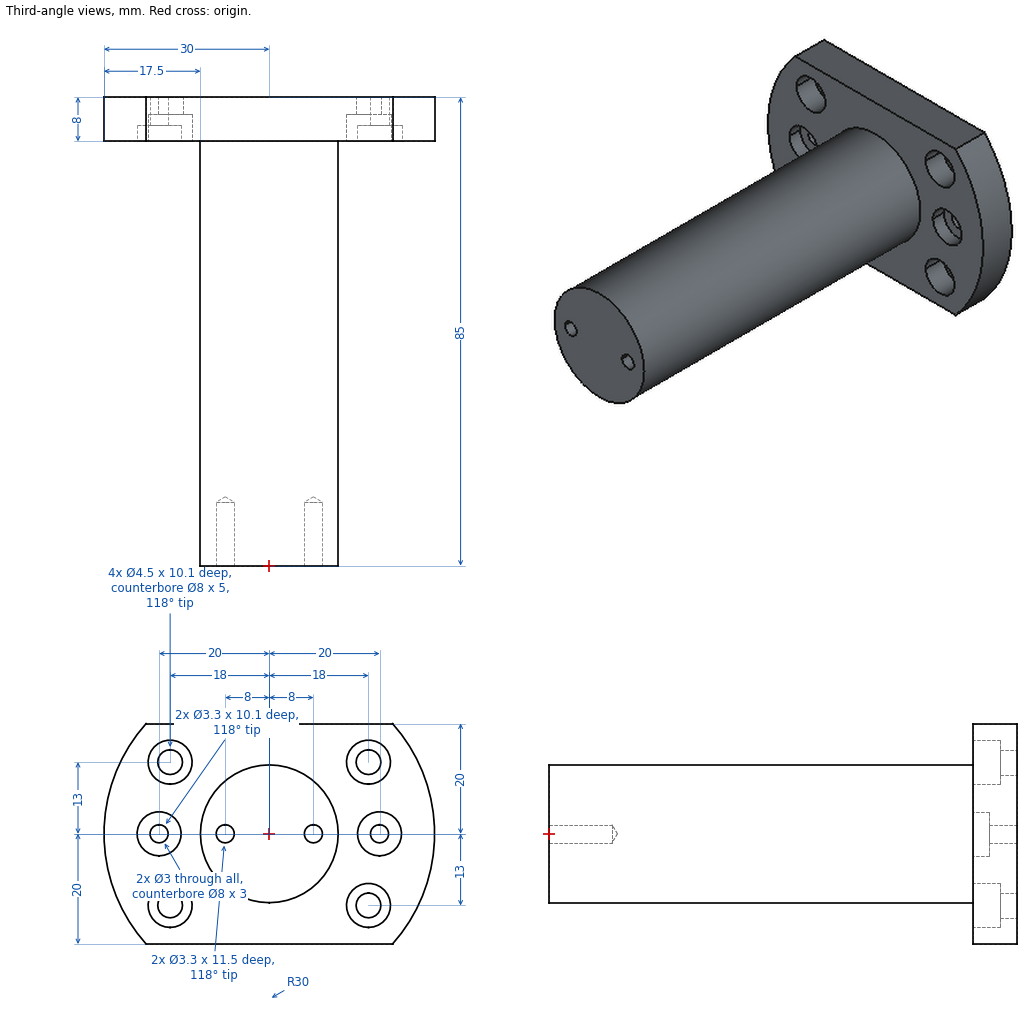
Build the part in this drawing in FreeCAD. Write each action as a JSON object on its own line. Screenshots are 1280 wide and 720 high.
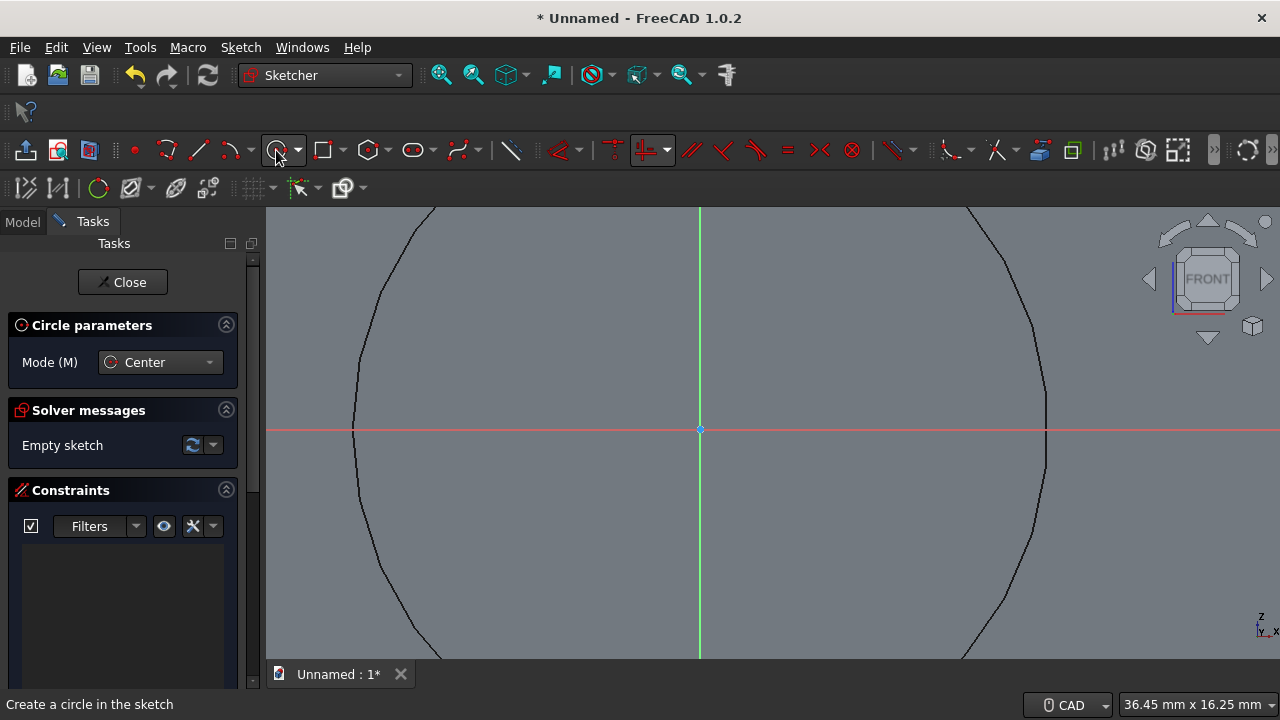
{"action": "left_click", "coordinate": [478, 430]}
{"action": "mouse_move", "coordinate": [510, 397]}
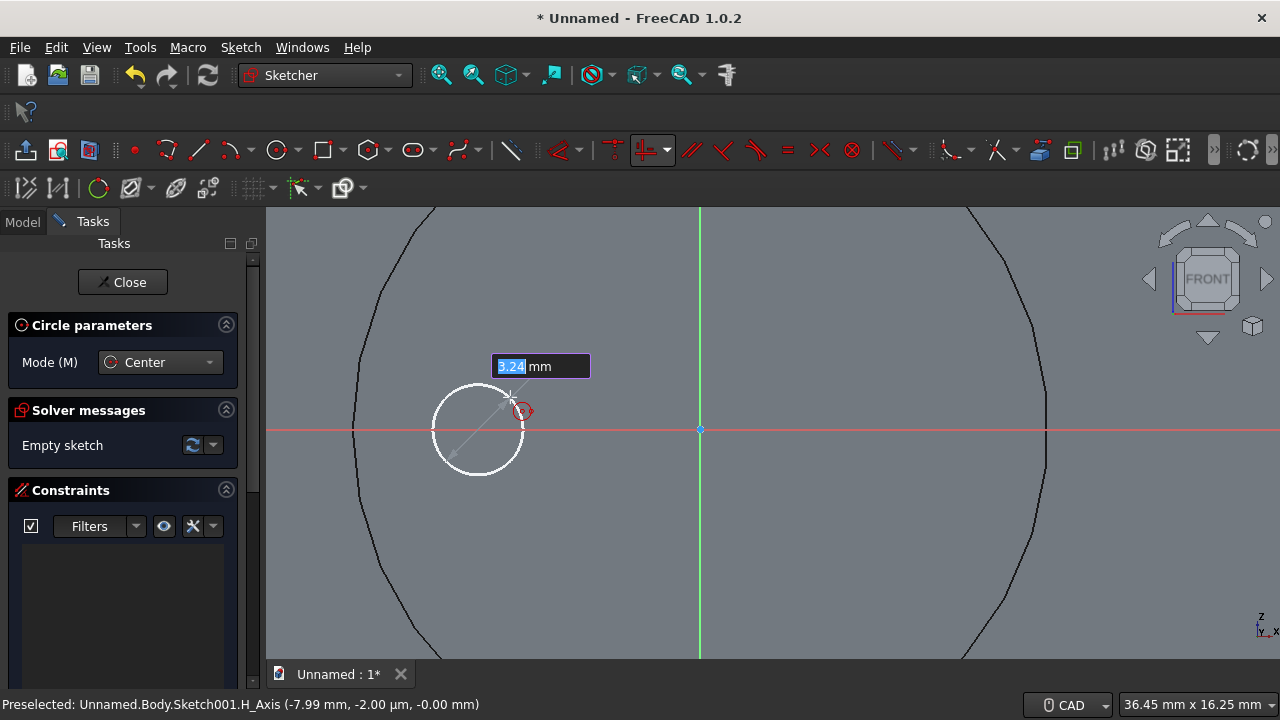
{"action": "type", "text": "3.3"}
{"action": "key", "text": "Return"}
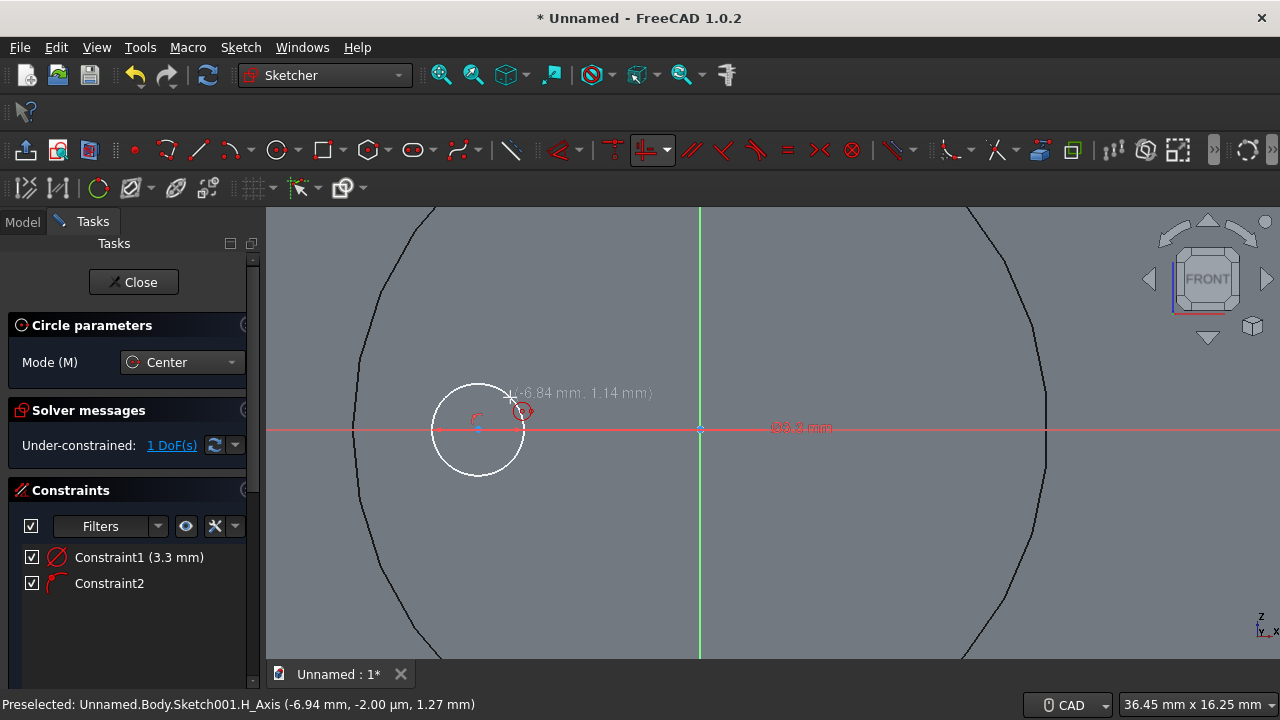
{"action": "left_click", "coordinate": [923, 430]}
{"action": "mouse_move", "coordinate": [955, 397]}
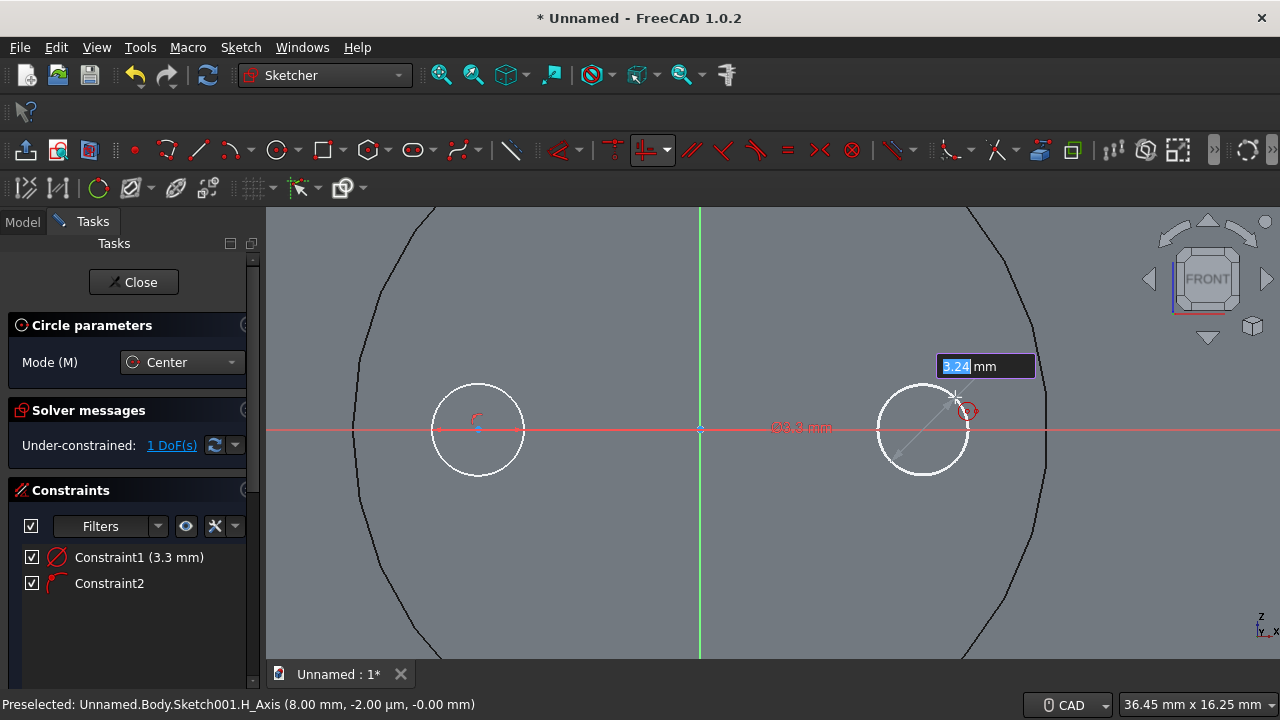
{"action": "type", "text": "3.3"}
{"action": "key", "text": "Return"}
{"action": "key", "text": "Escape"}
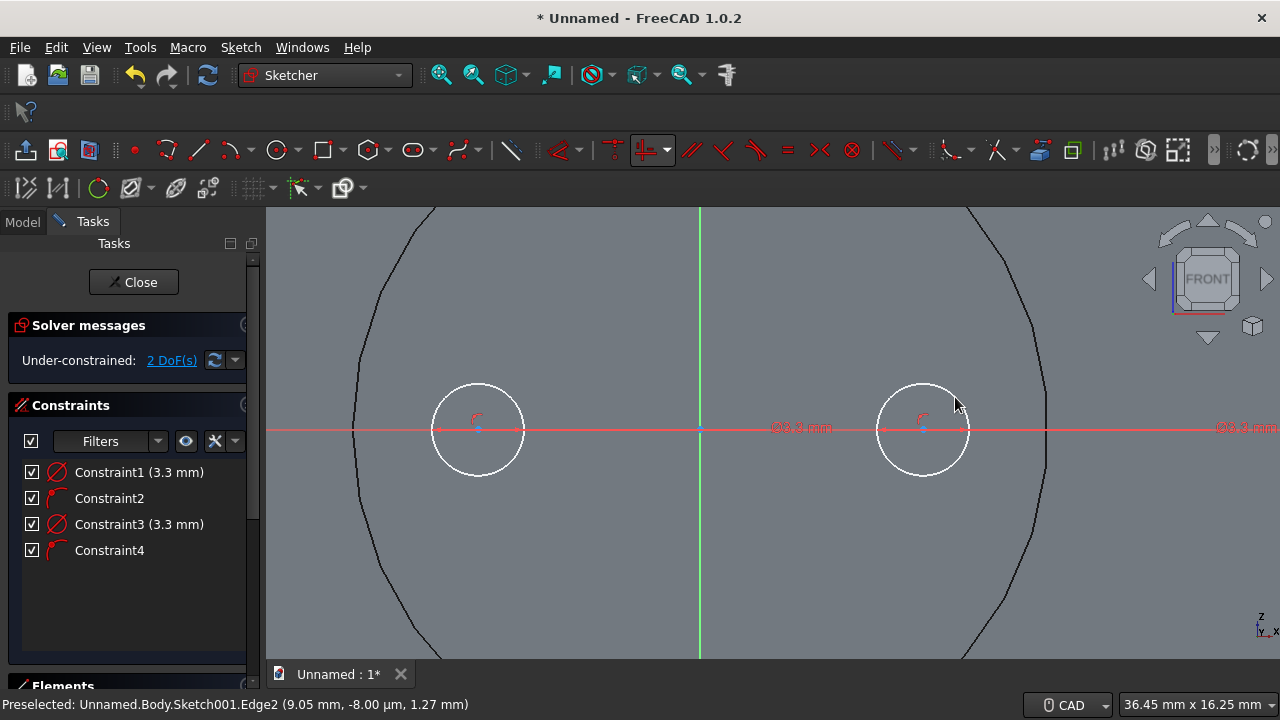
{"action": "left_click", "coordinate": [558, 150]}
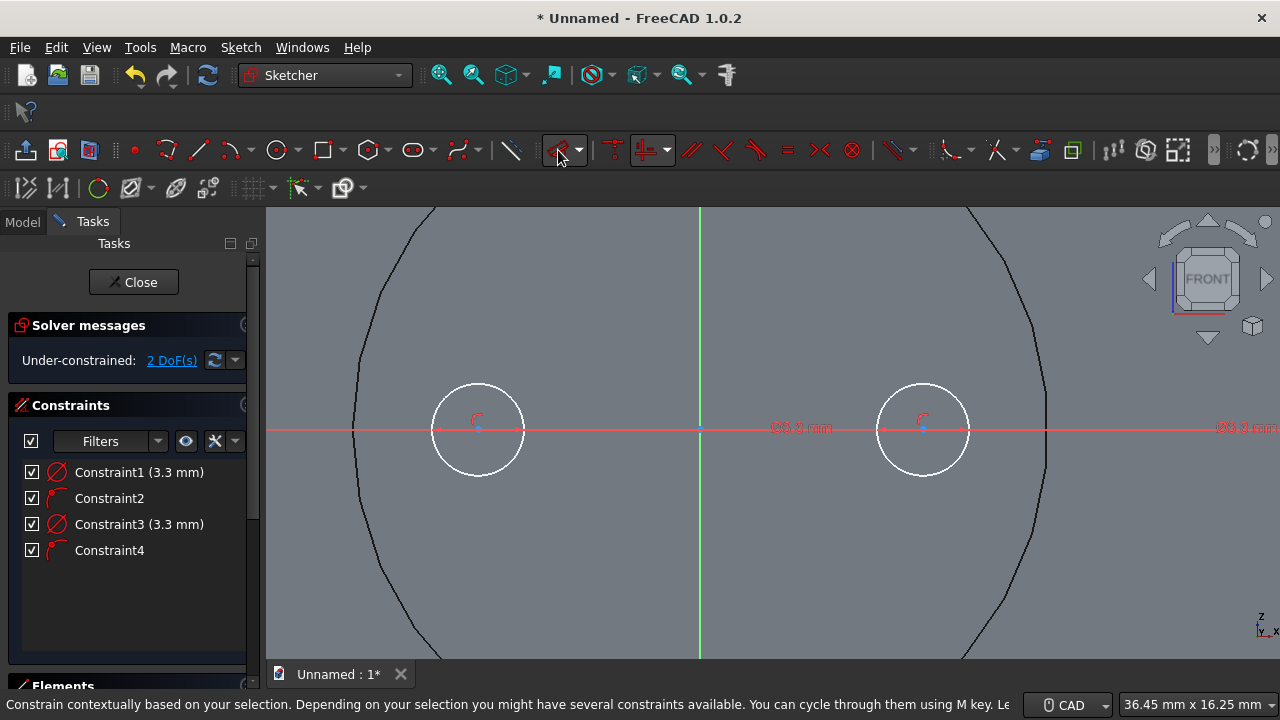
{"action": "left_click", "coordinate": [478, 430]}
{"action": "left_click", "coordinate": [589, 464]}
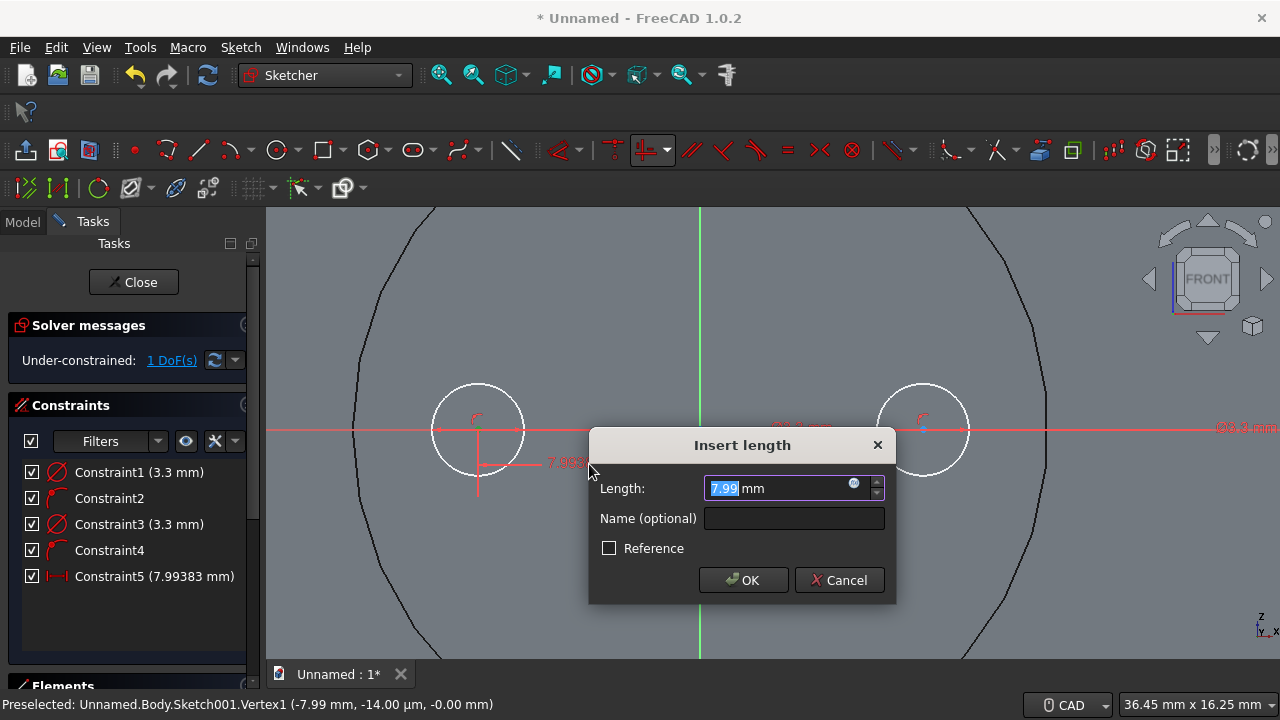
{"action": "type", "text": "8"}
{"action": "key", "text": "Return"}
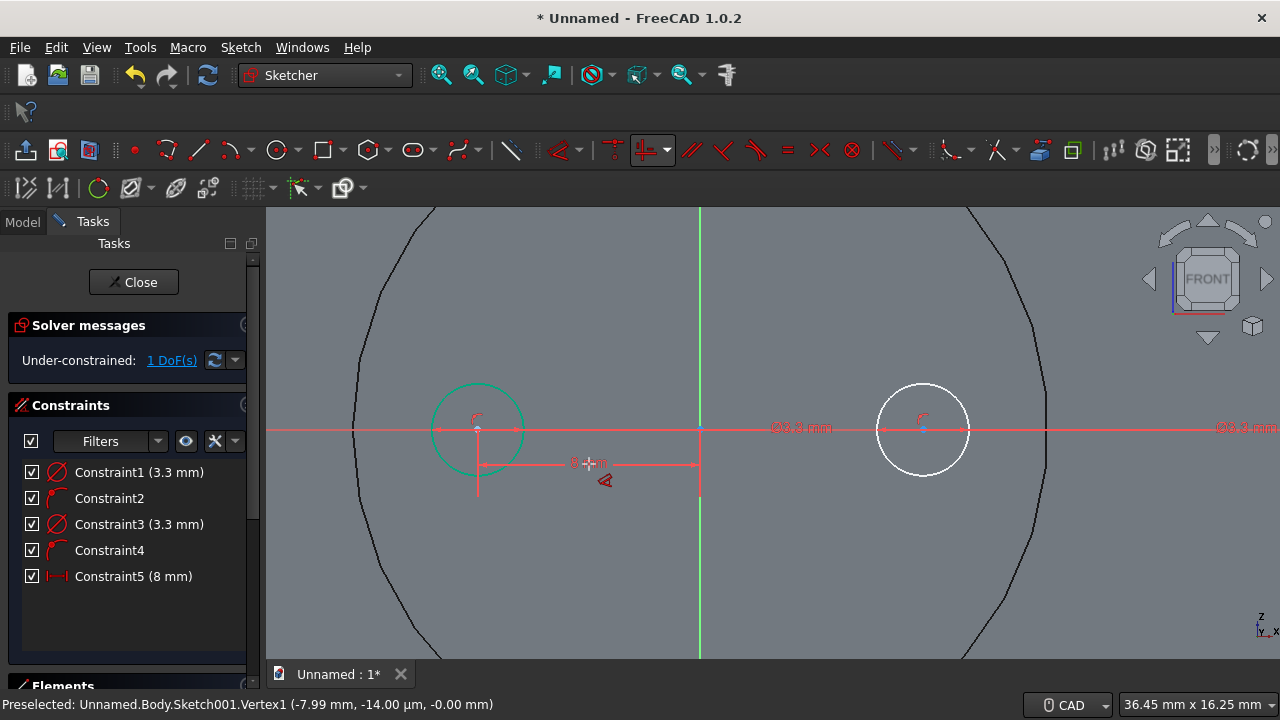
{"action": "left_click", "coordinate": [923, 430]}
{"action": "left_click", "coordinate": [812, 464]}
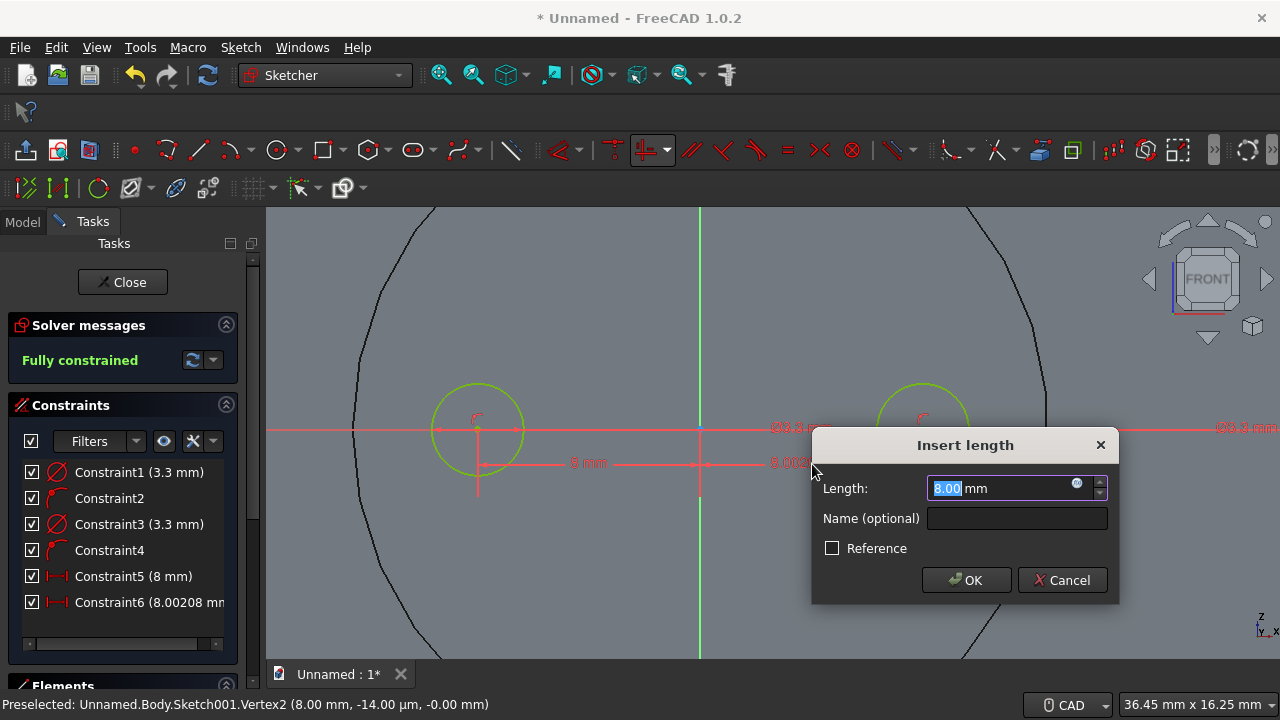
{"action": "type", "text": "8"}
{"action": "key", "text": "Return"}
{"action": "key", "text": "Escape"}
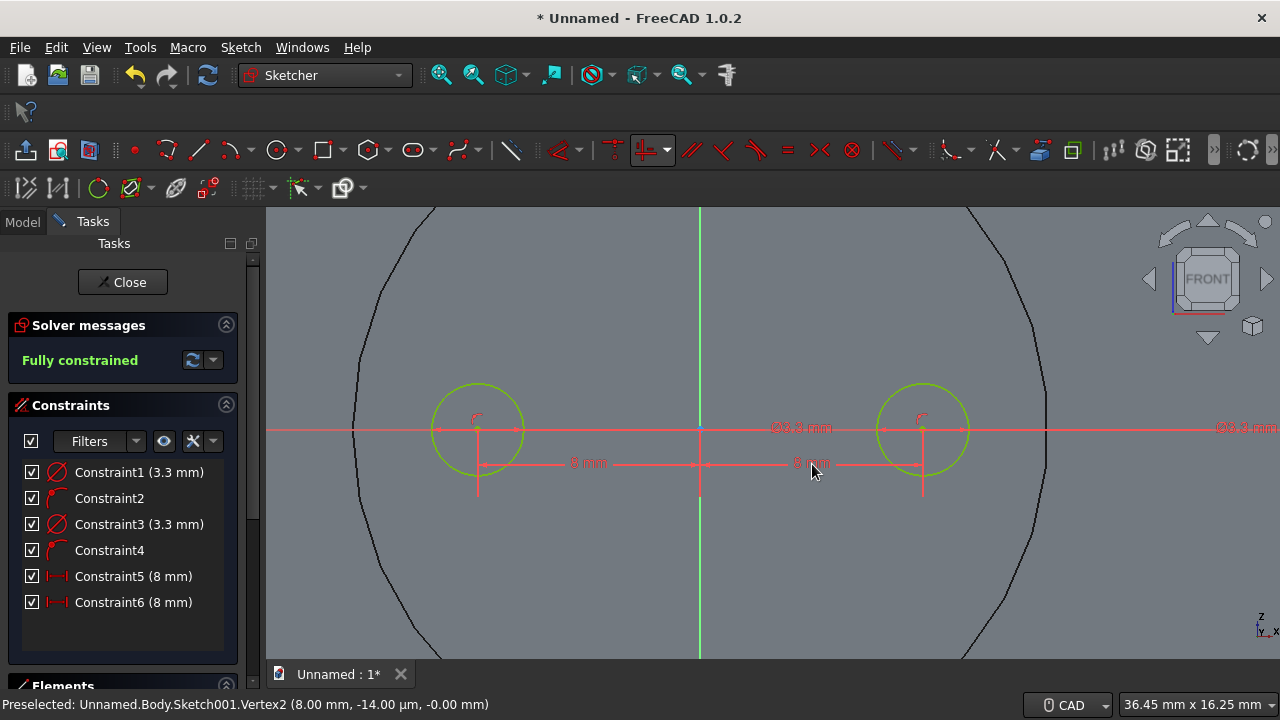
{"action": "left_click", "coordinate": [123, 282]}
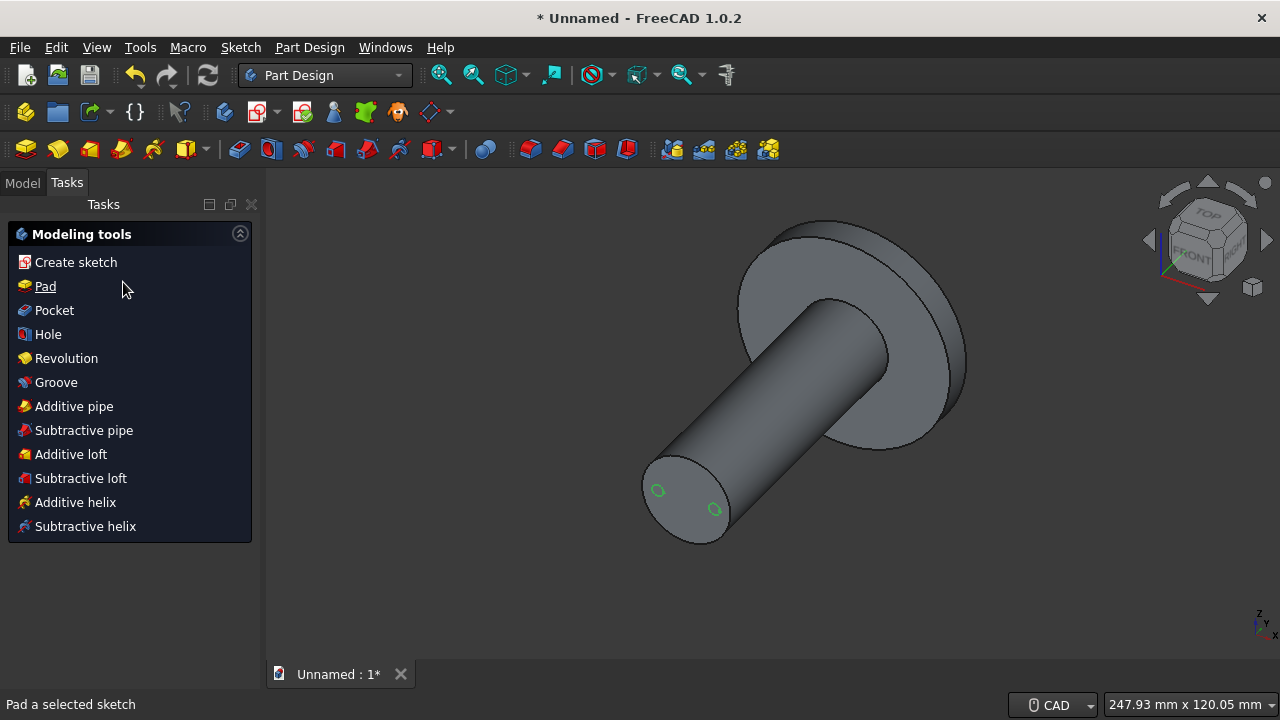
{"action": "left_click", "coordinate": [272, 150]}